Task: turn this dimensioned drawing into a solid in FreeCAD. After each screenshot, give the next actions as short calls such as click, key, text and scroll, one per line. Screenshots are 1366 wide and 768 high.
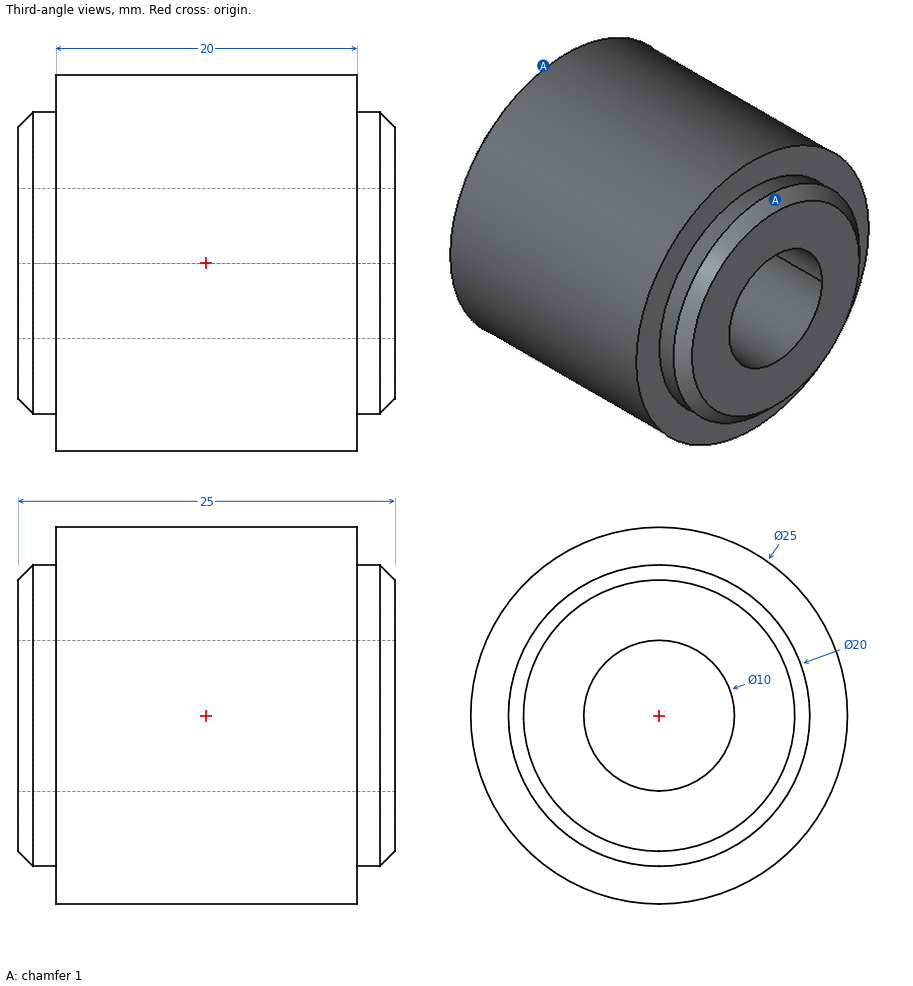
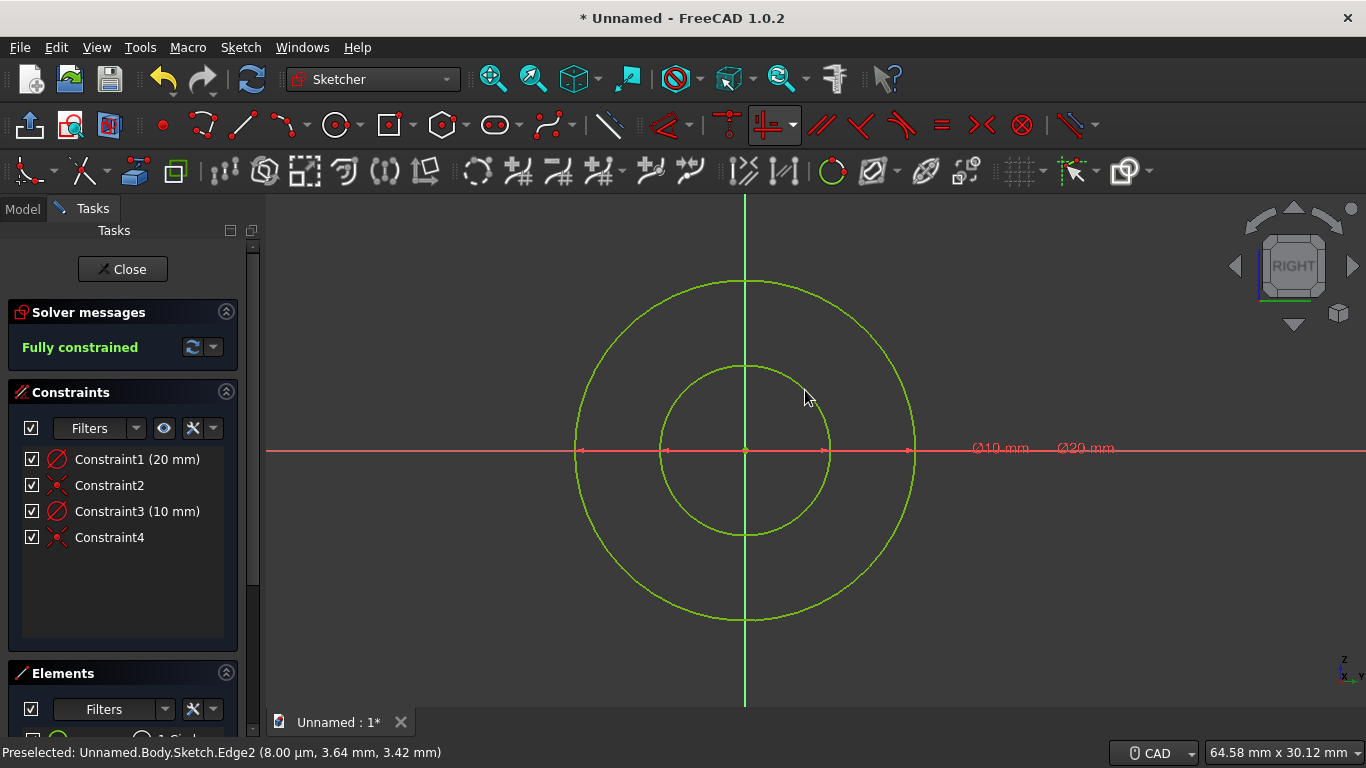
click(123, 269)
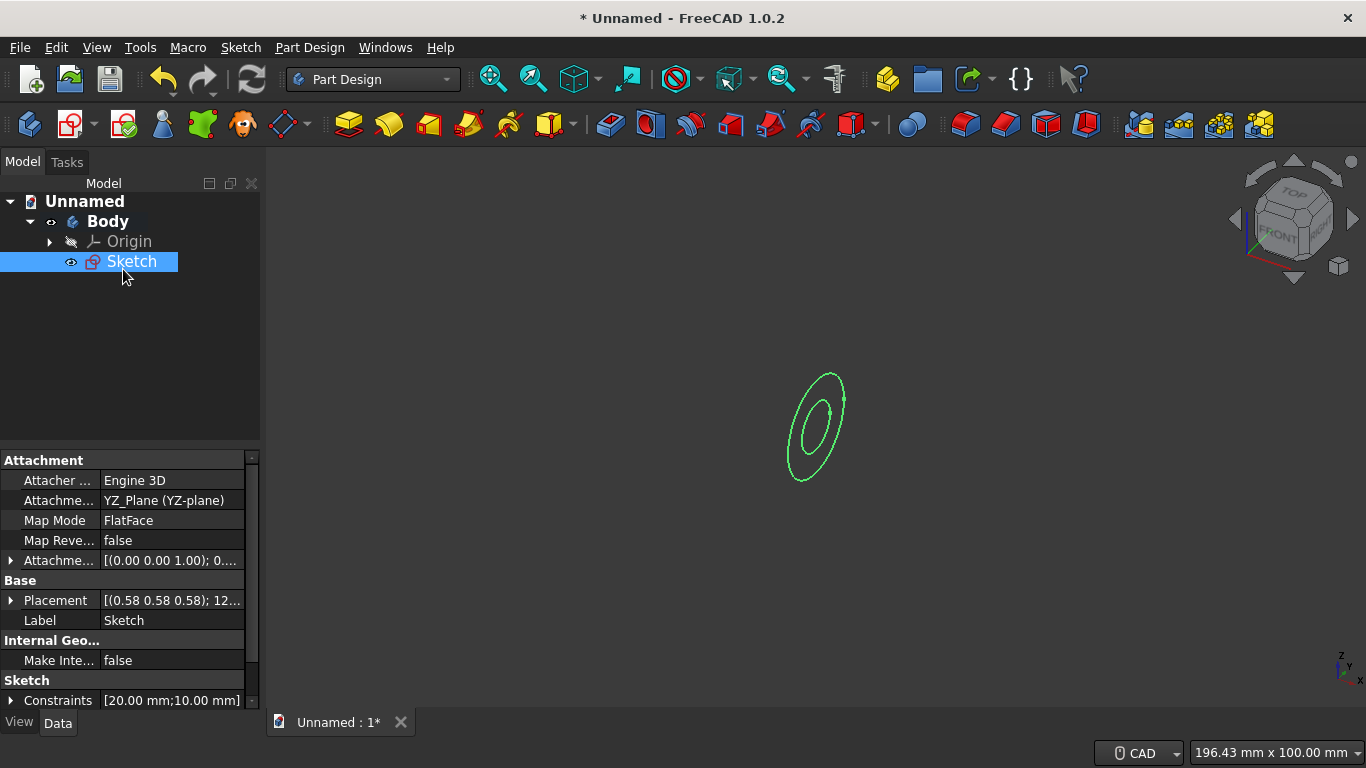
click(350, 124)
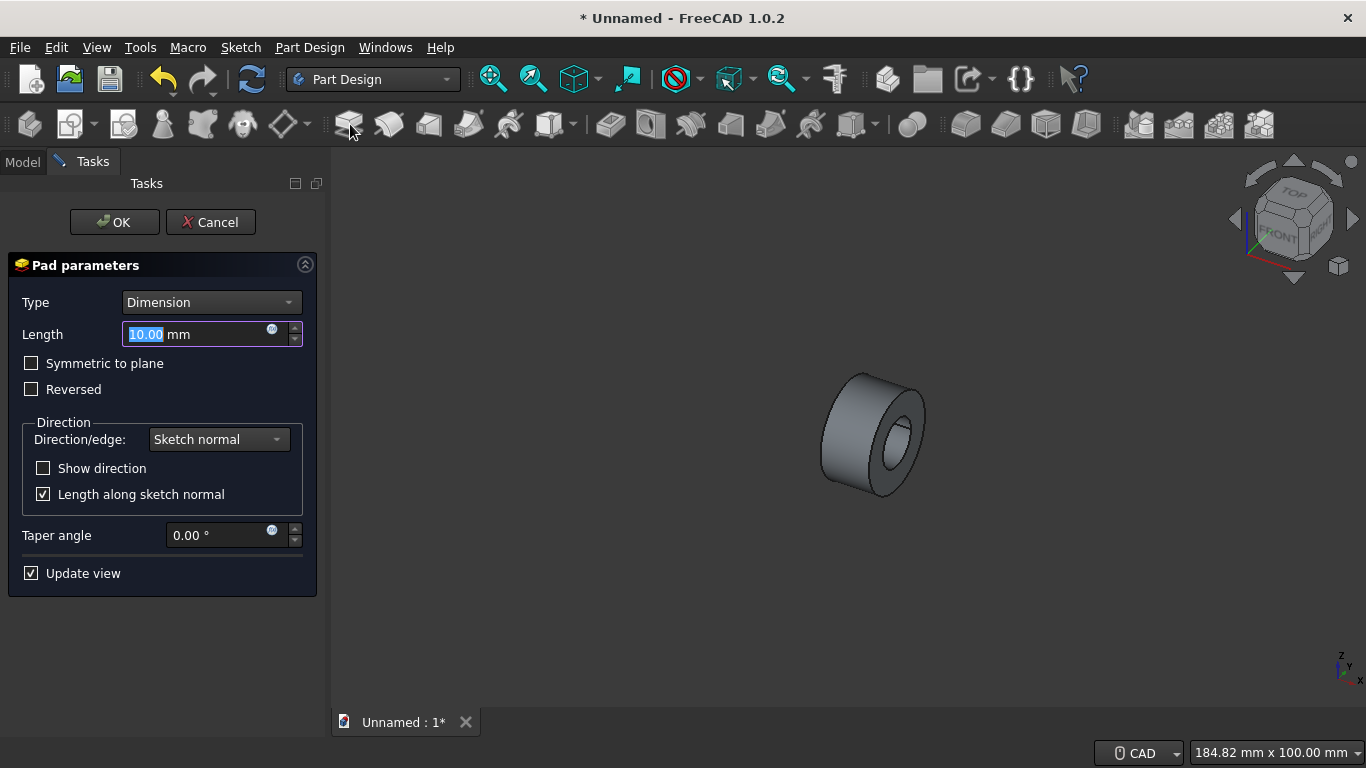
text(25)
key(Tab)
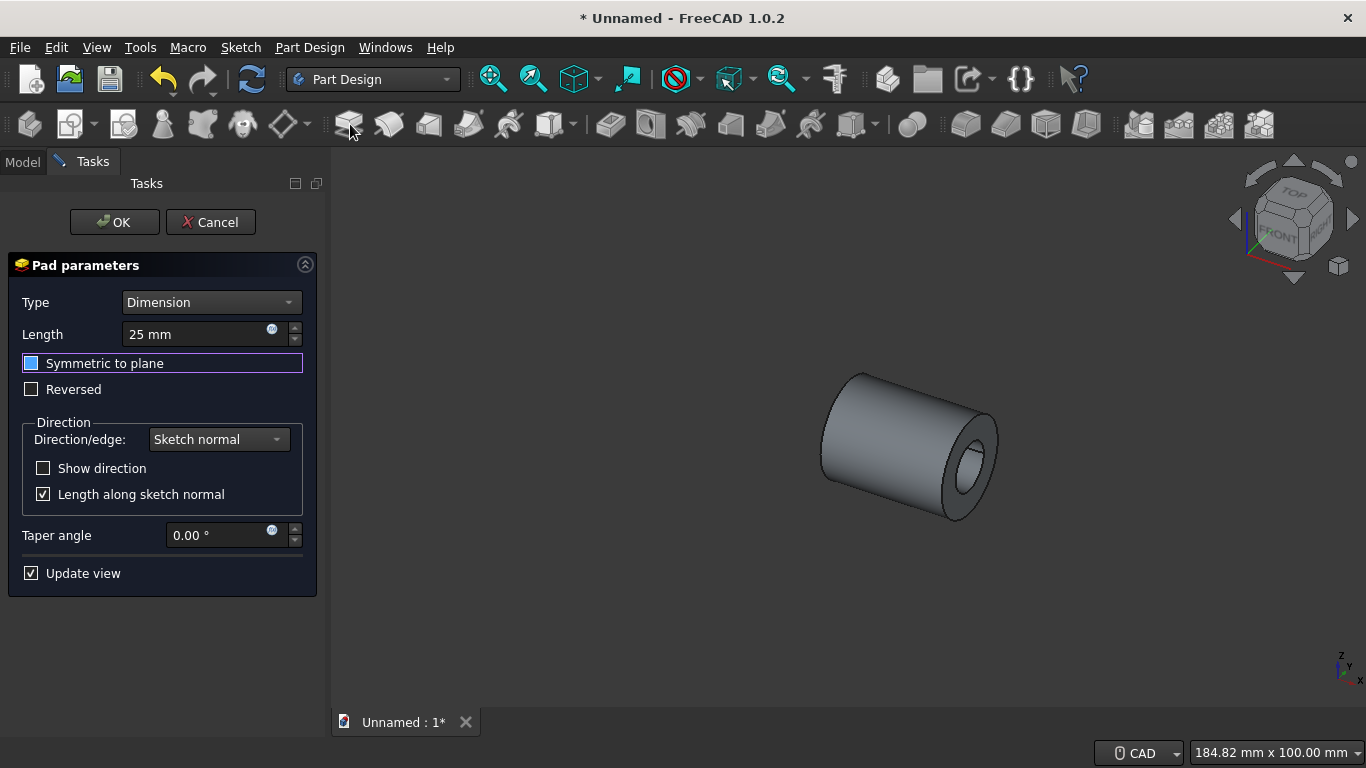
click(30, 363)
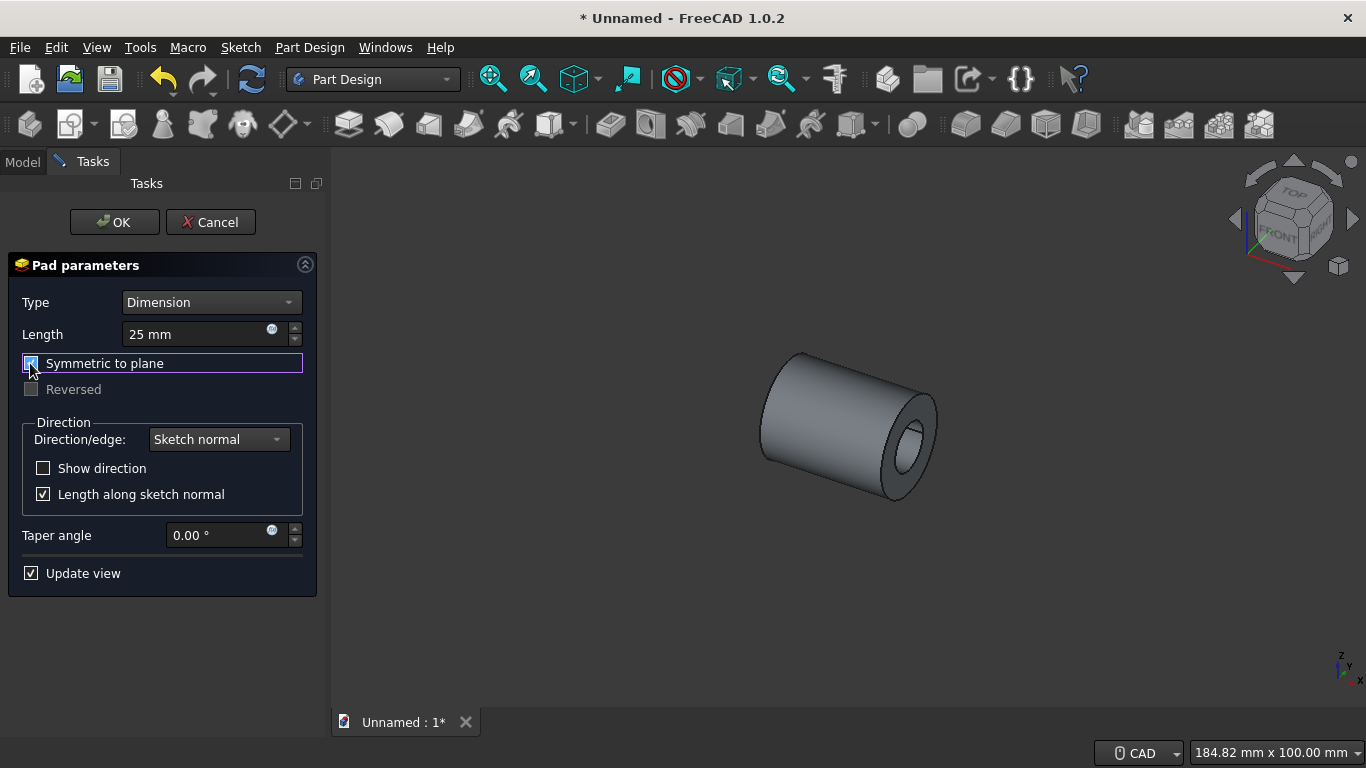
click(115, 222)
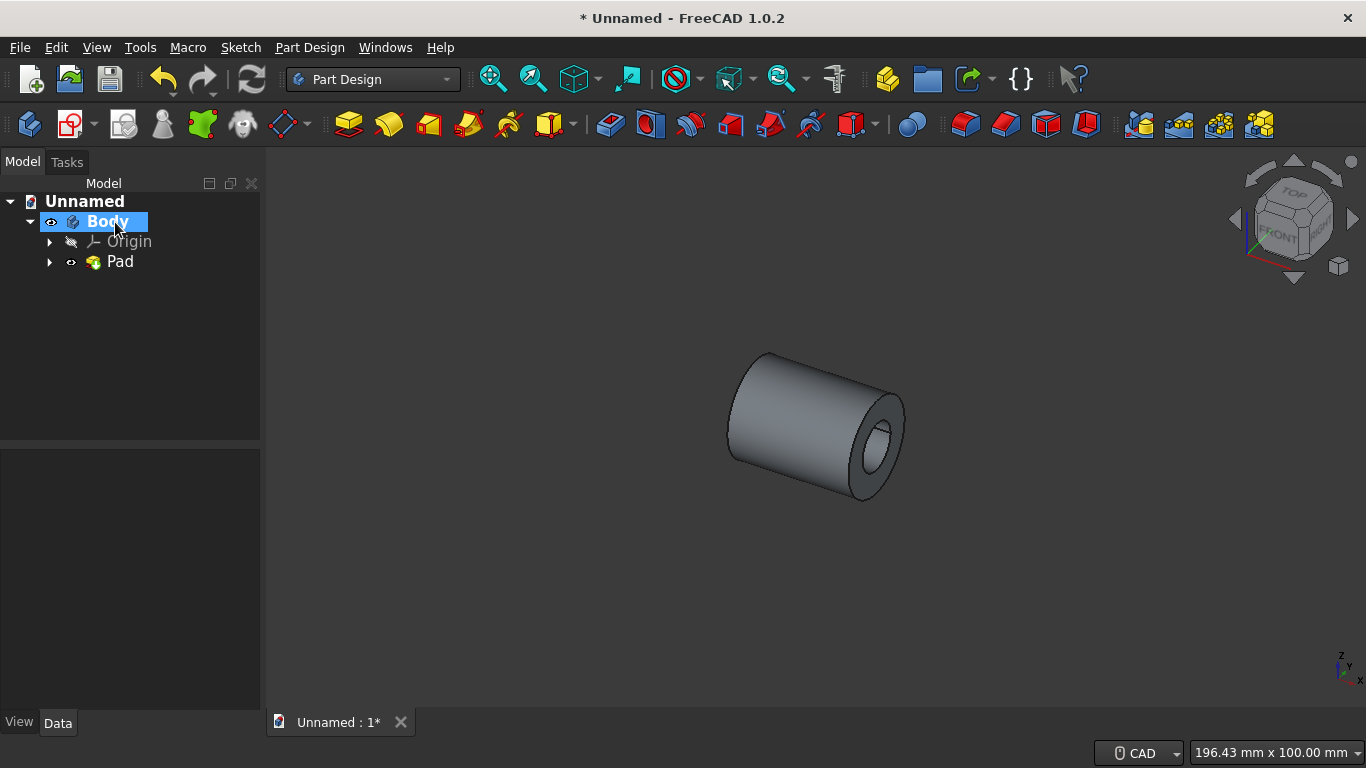
key(v)
key(f)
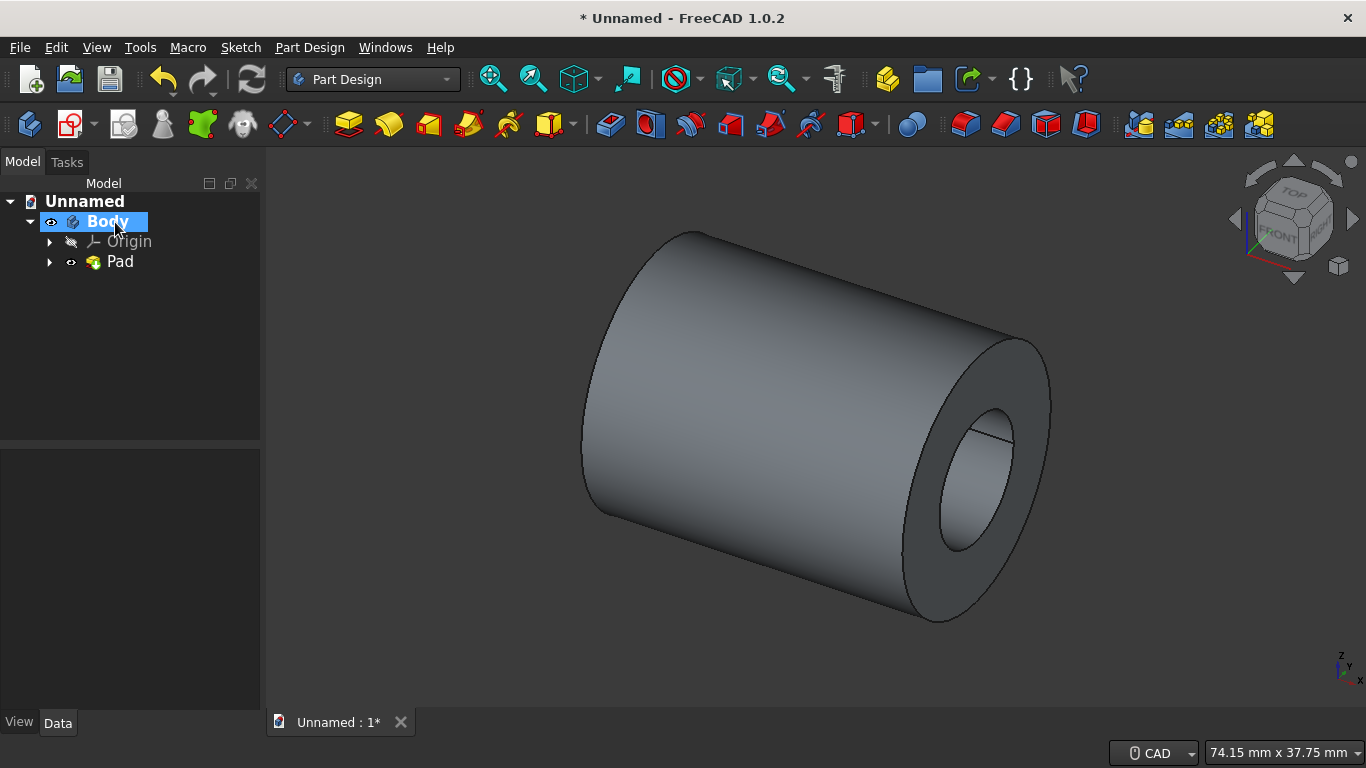
click(70, 124)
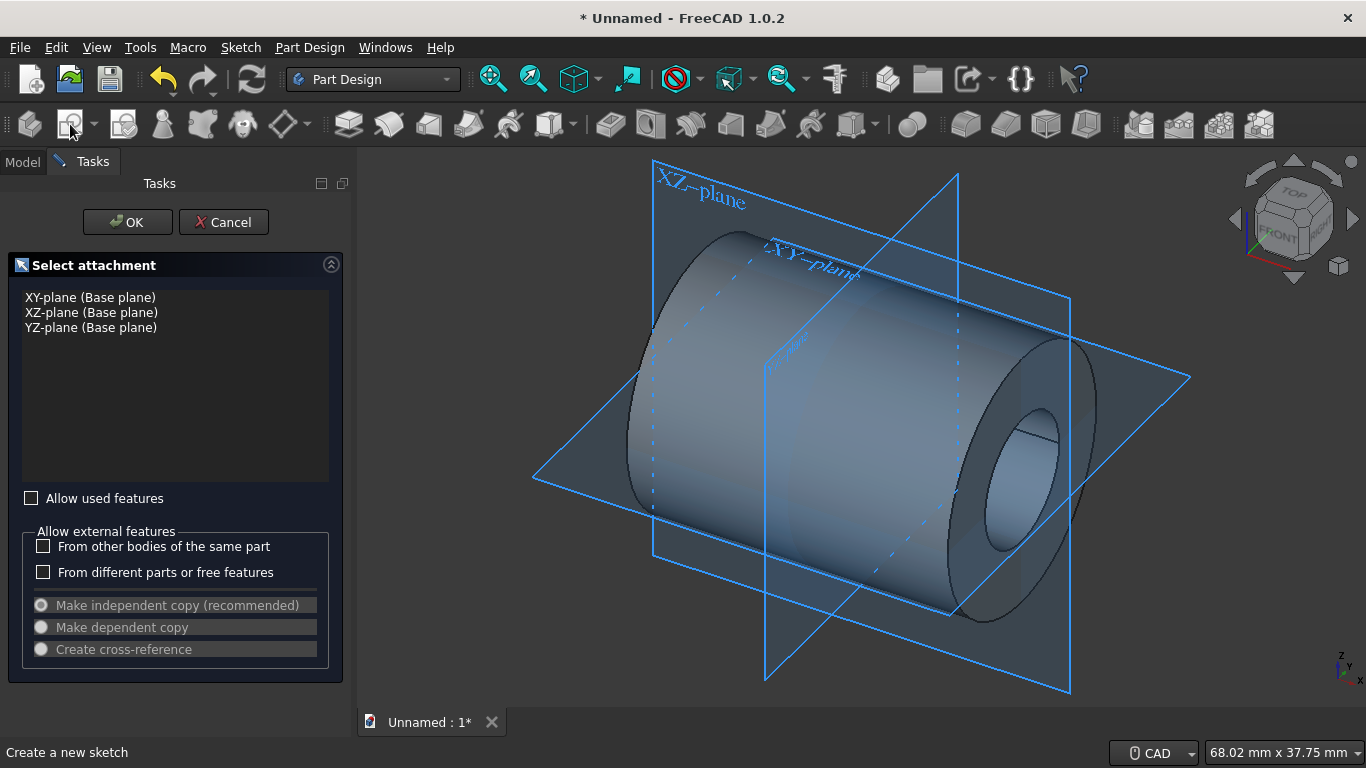
click(82, 328)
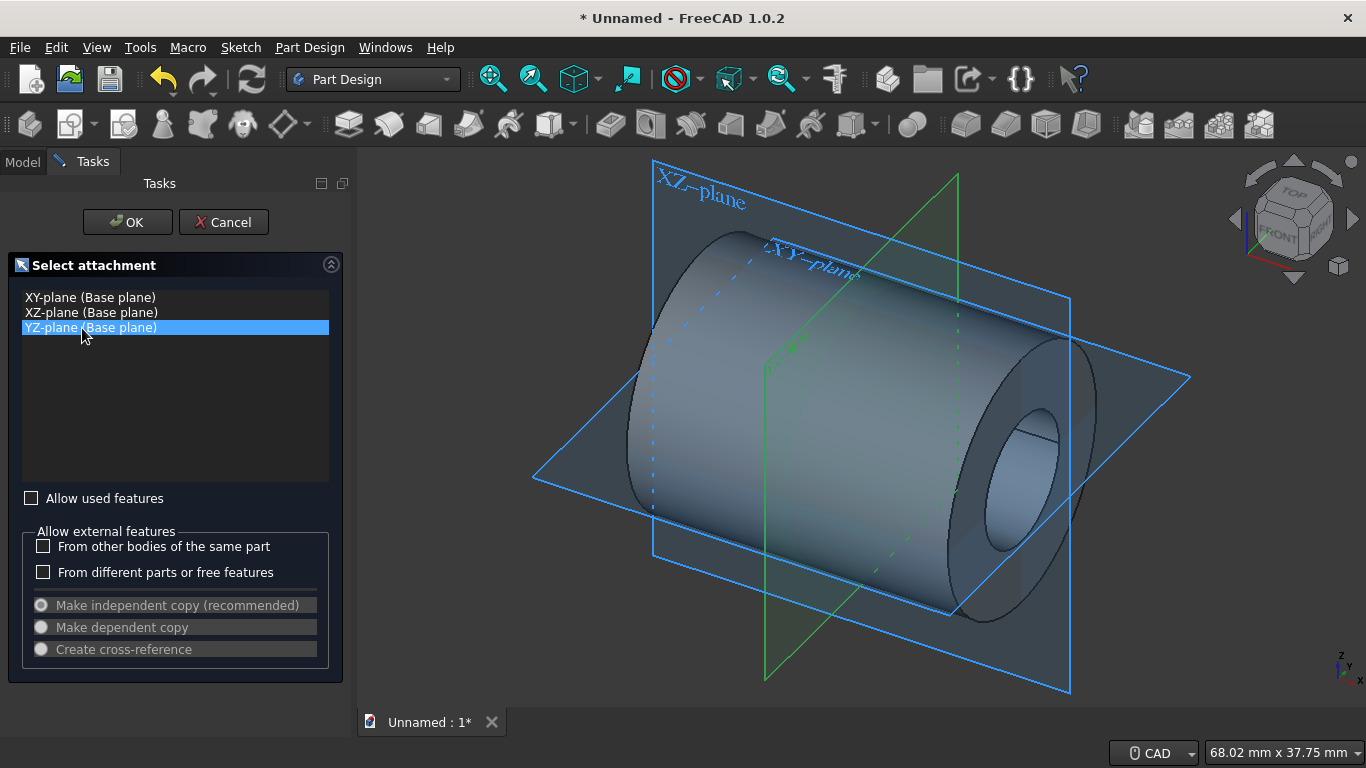
click(128, 222)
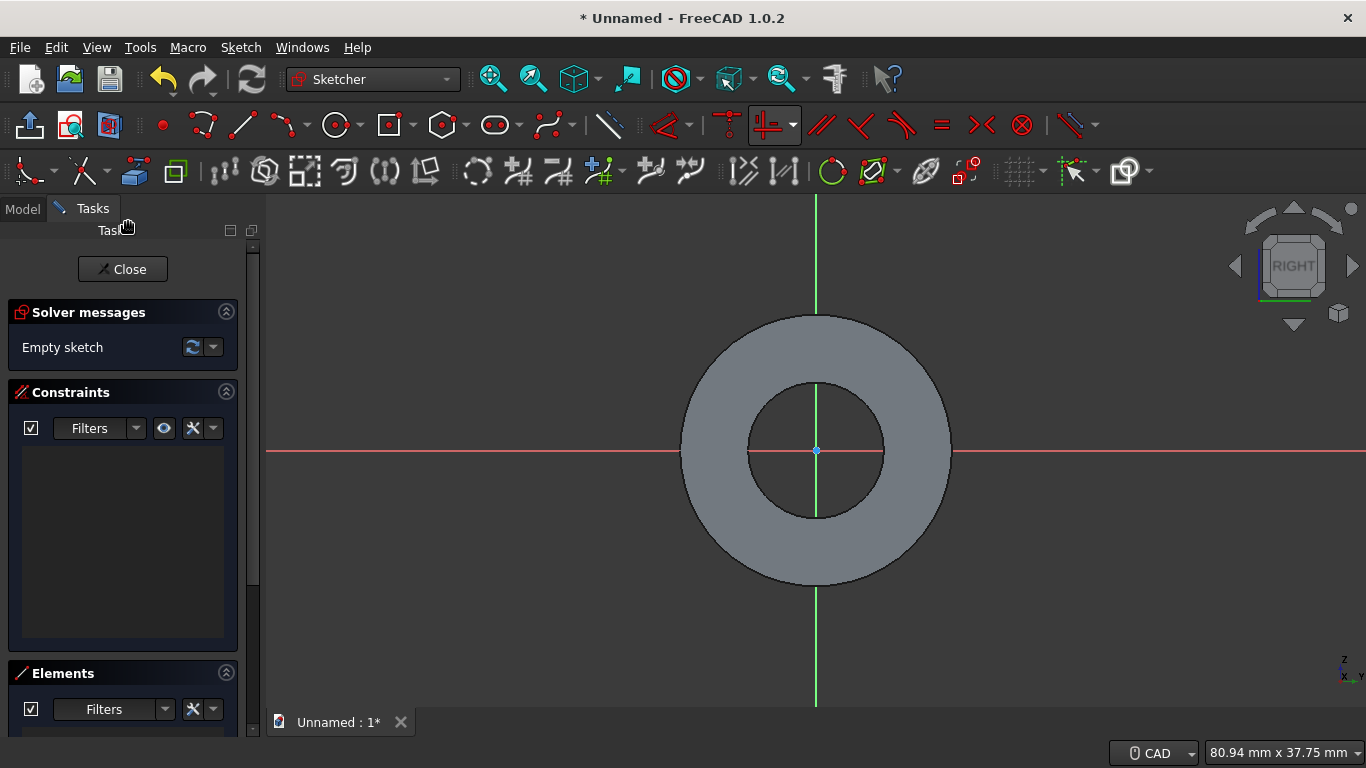
key(q)
key(s)